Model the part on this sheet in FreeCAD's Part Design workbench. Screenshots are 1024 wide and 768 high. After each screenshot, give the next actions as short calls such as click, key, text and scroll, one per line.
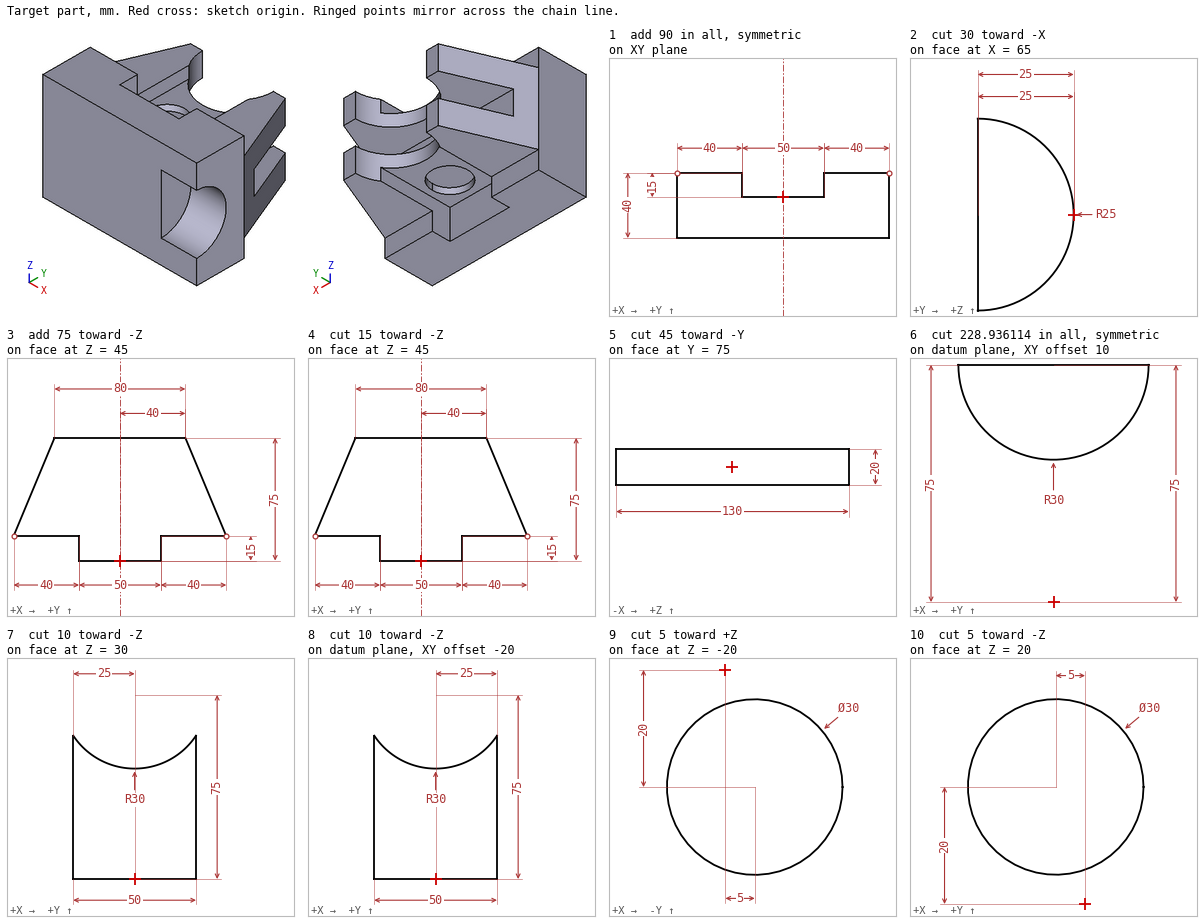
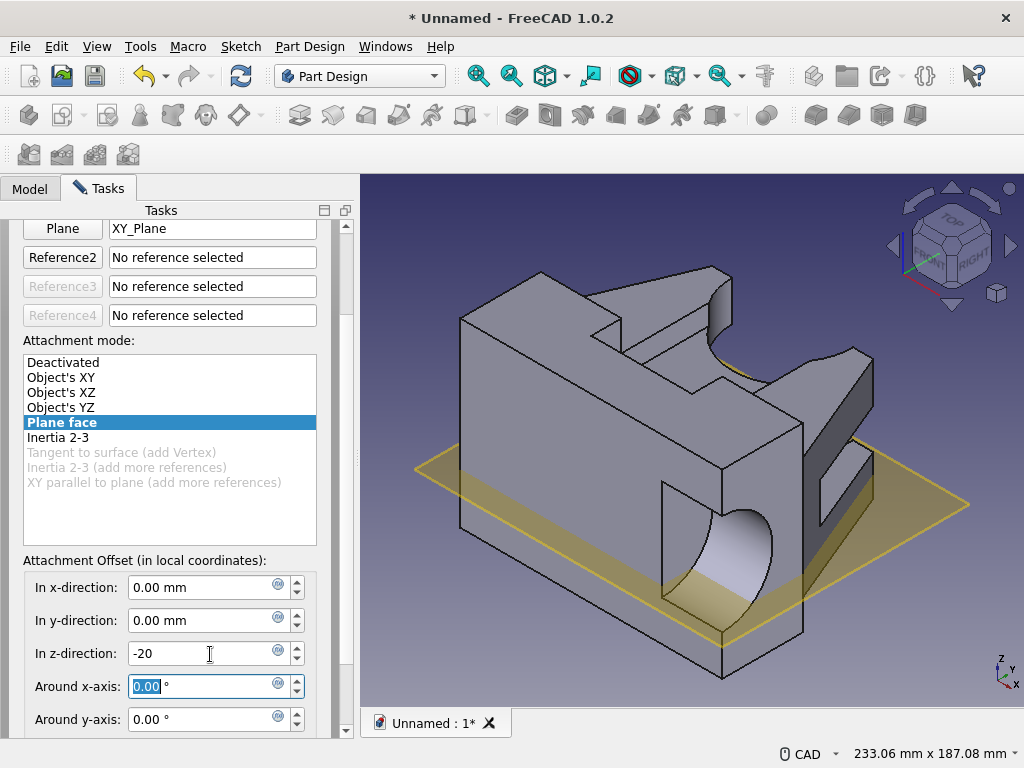
scroll(346, 479, up, 3)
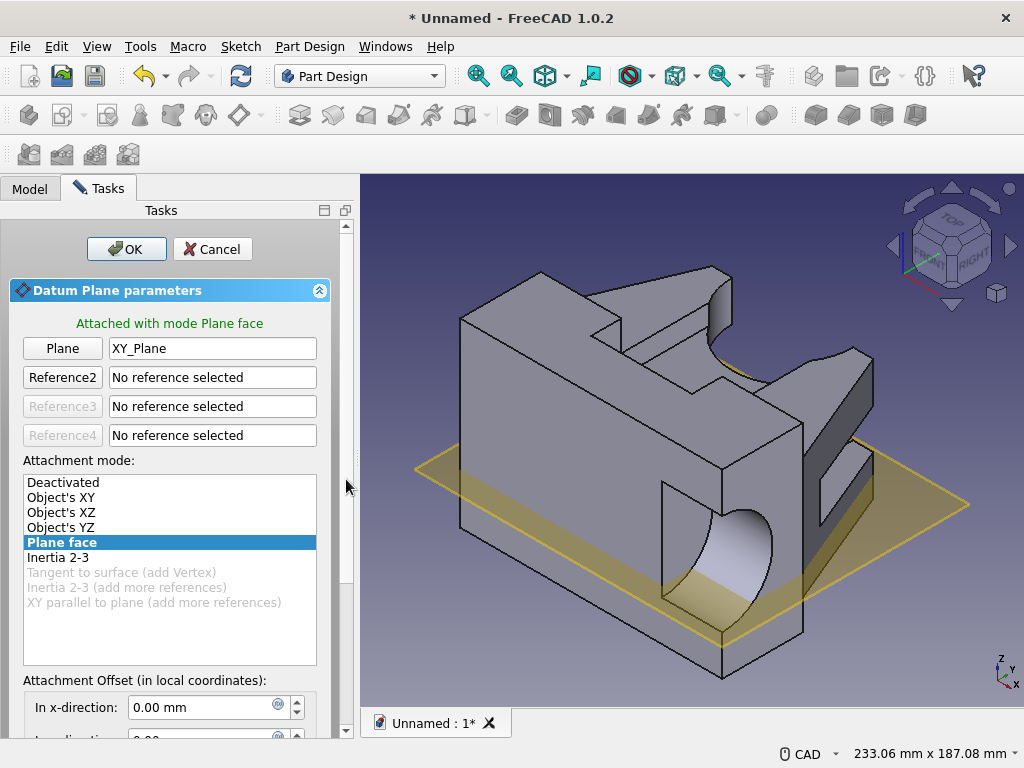
click(127, 249)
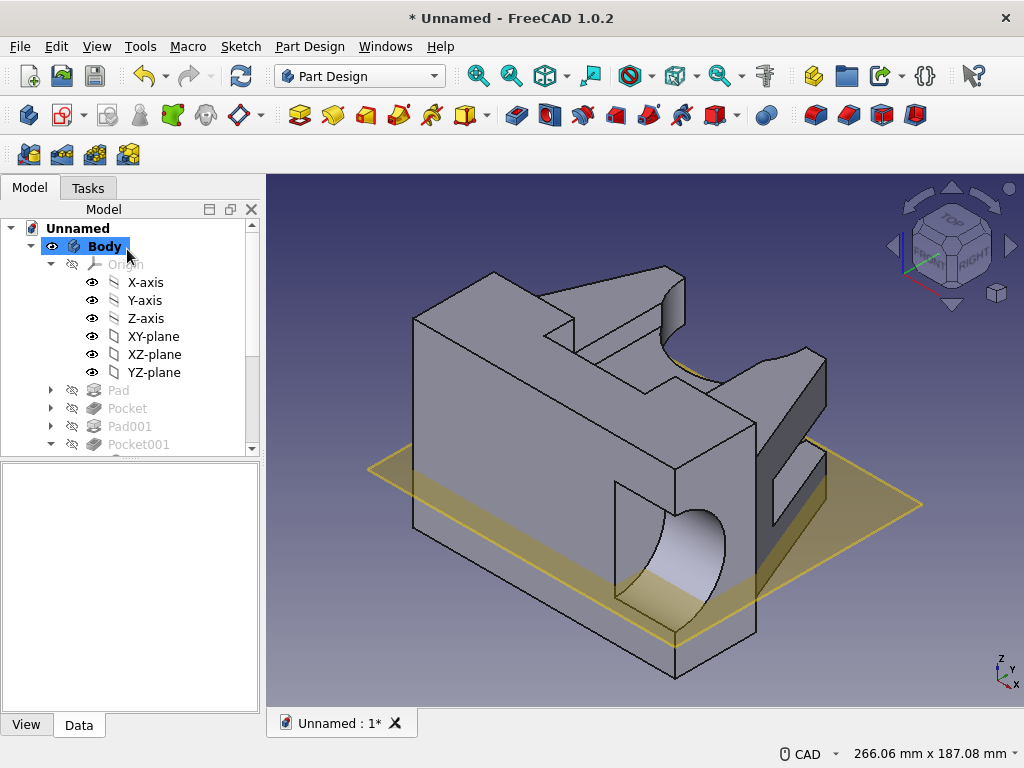
scroll(101, 332, down, 3)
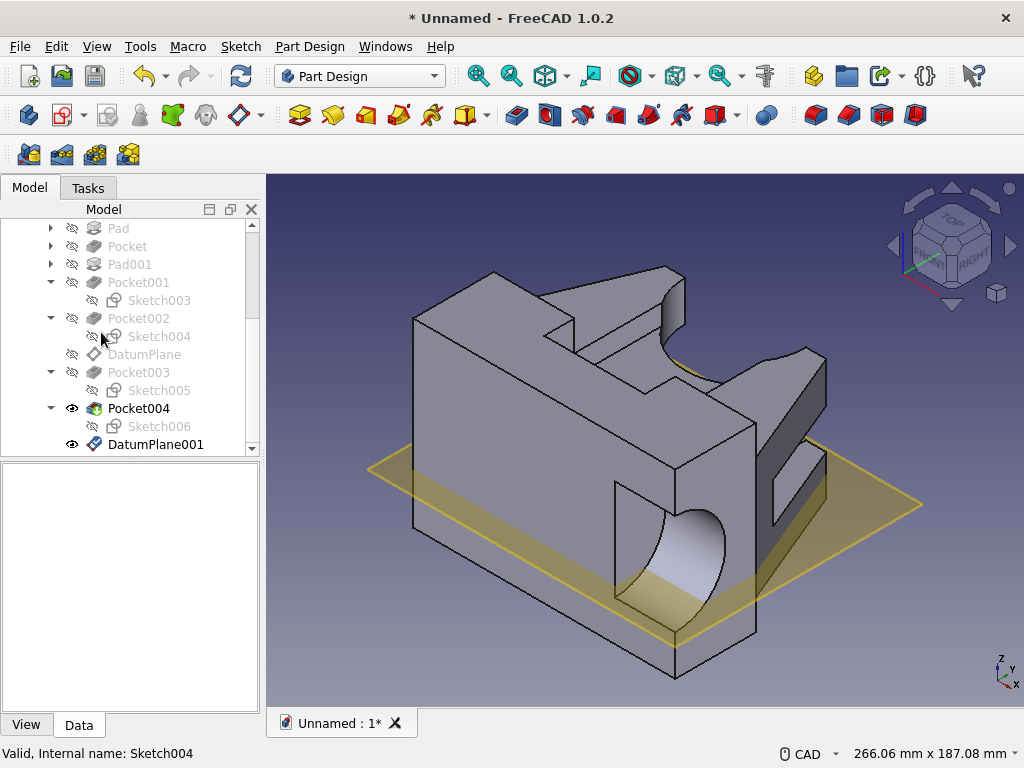
click(117, 444)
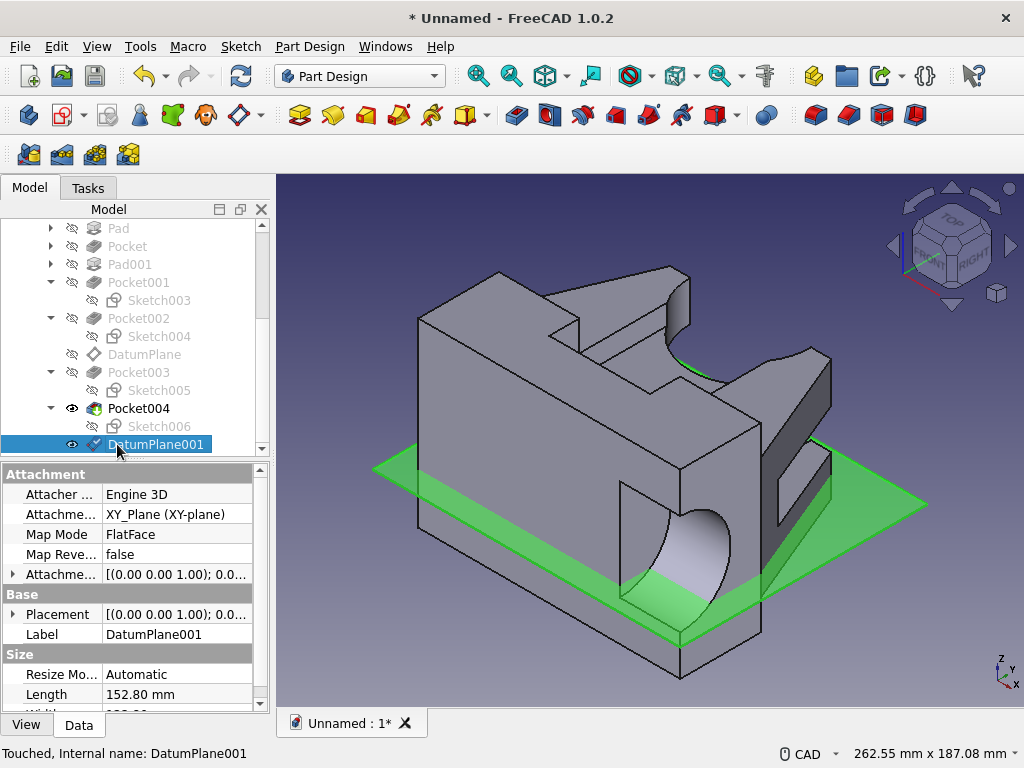
click(62, 116)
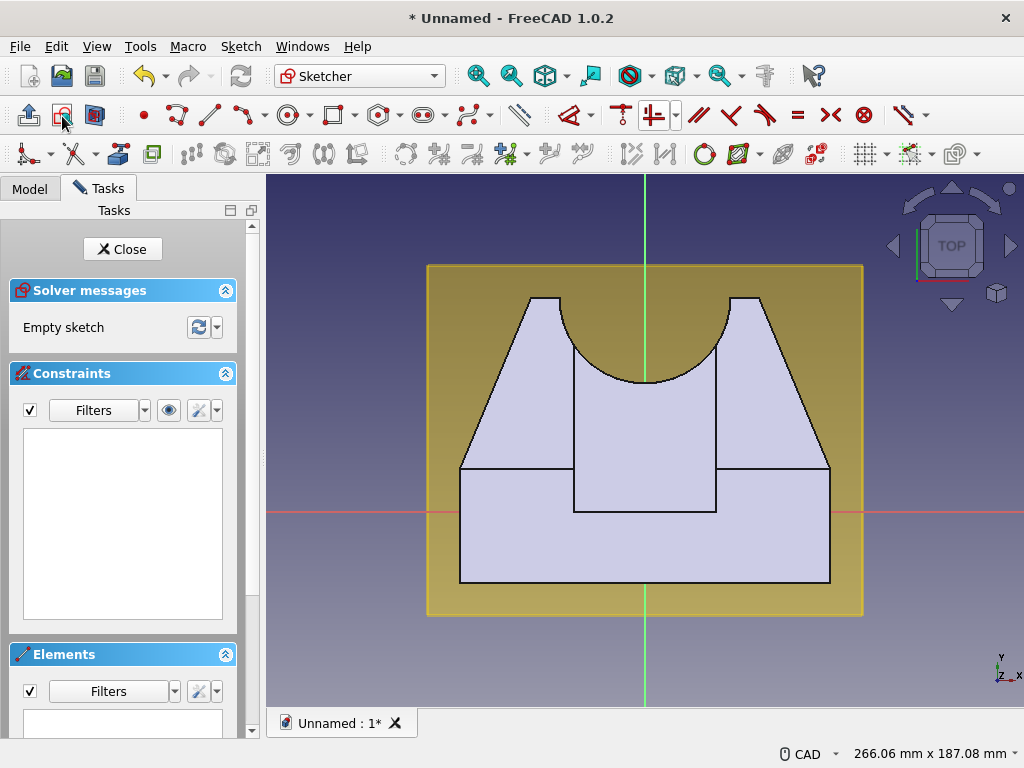
click(95, 116)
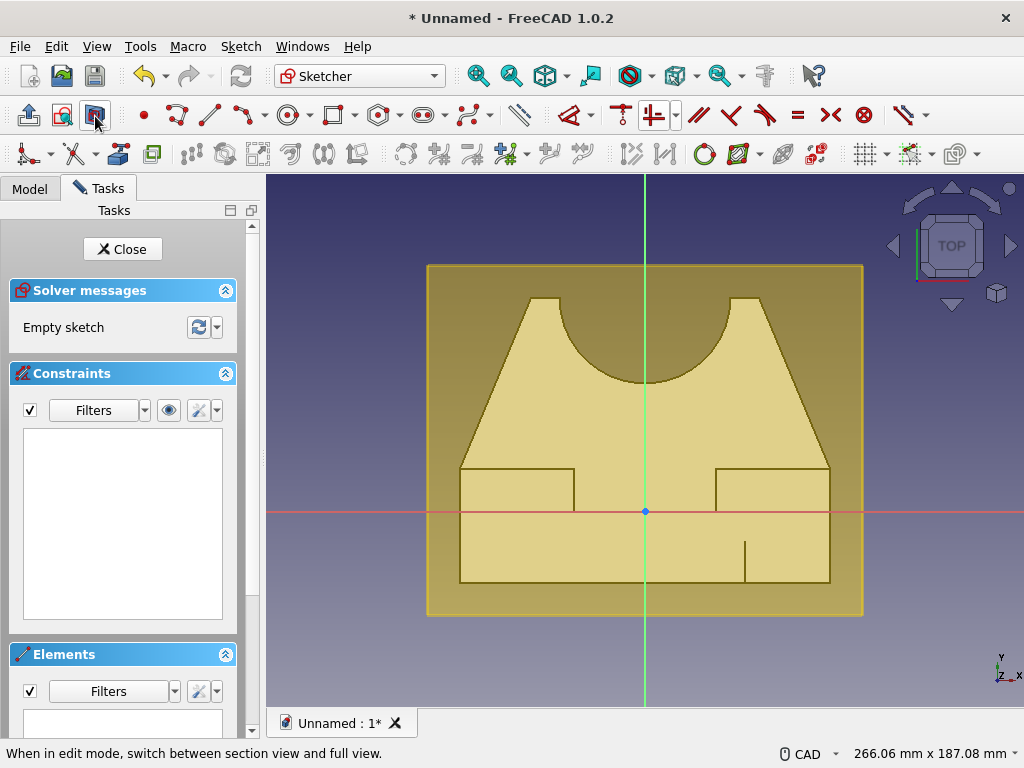
scroll(701, 419, up, 4)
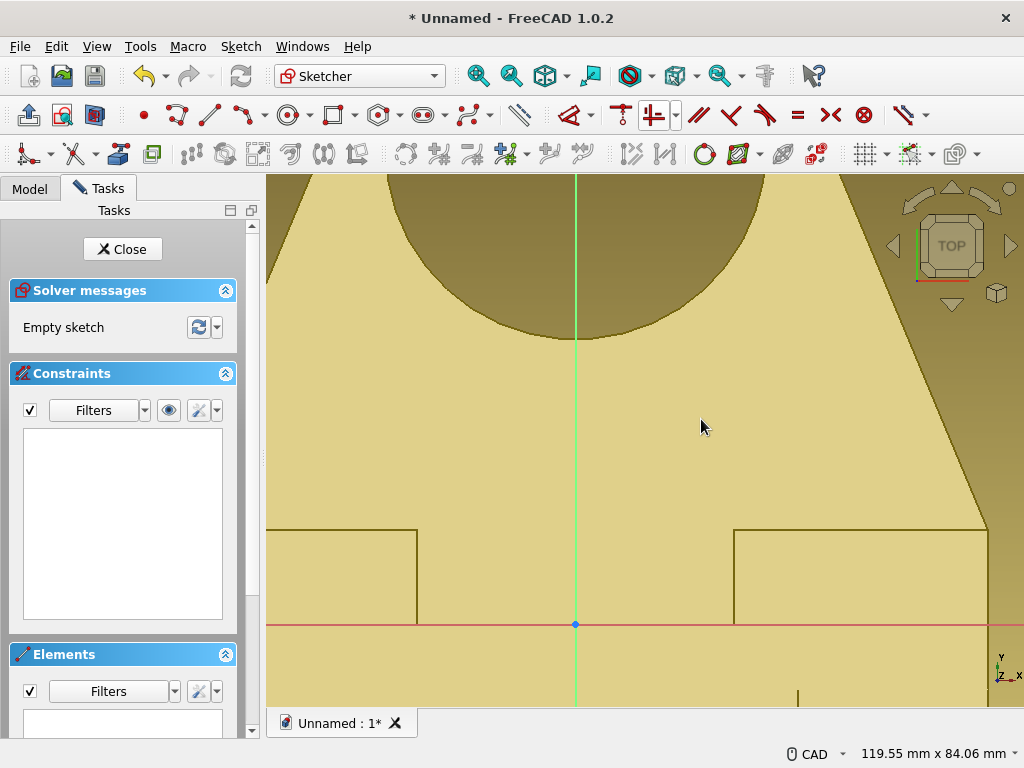
key(g)
key(m)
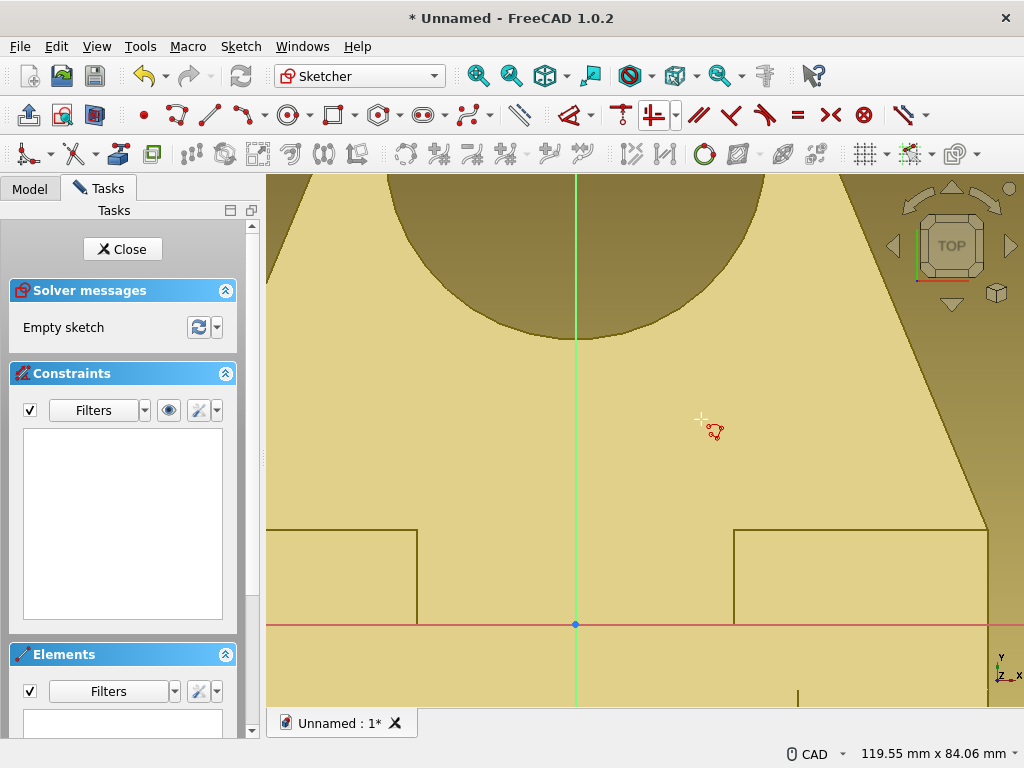
click(734, 254)
click(734, 625)
click(417, 616)
click(417, 254)
right_click(417, 254)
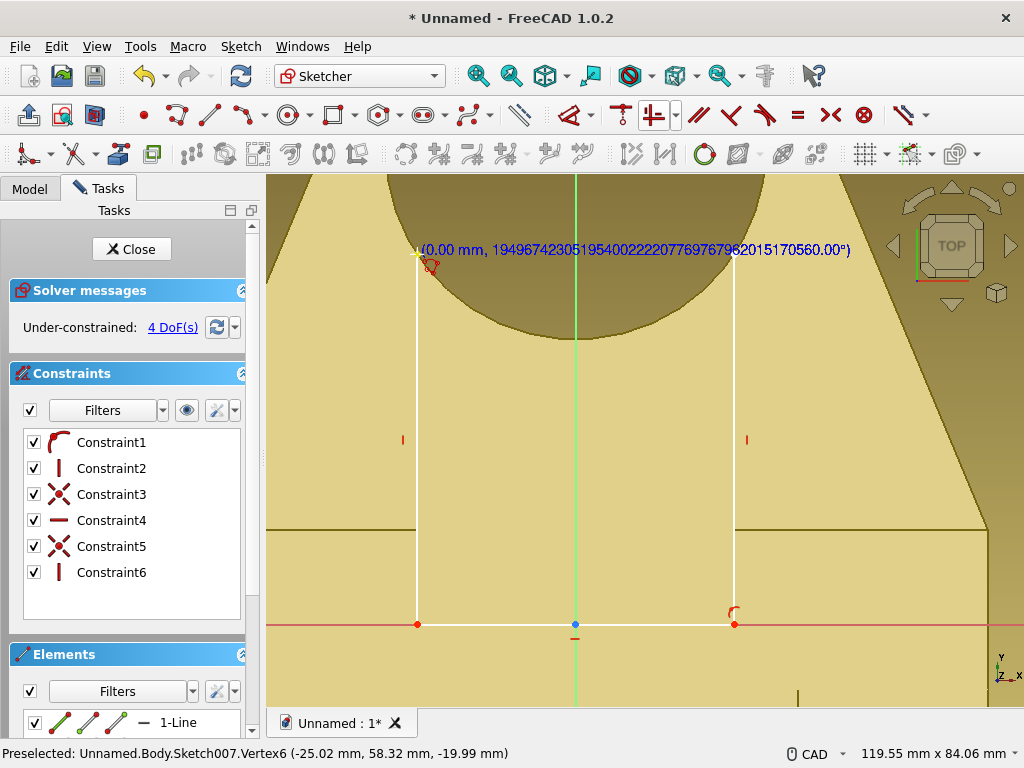
key(g)
key(3)
key(a)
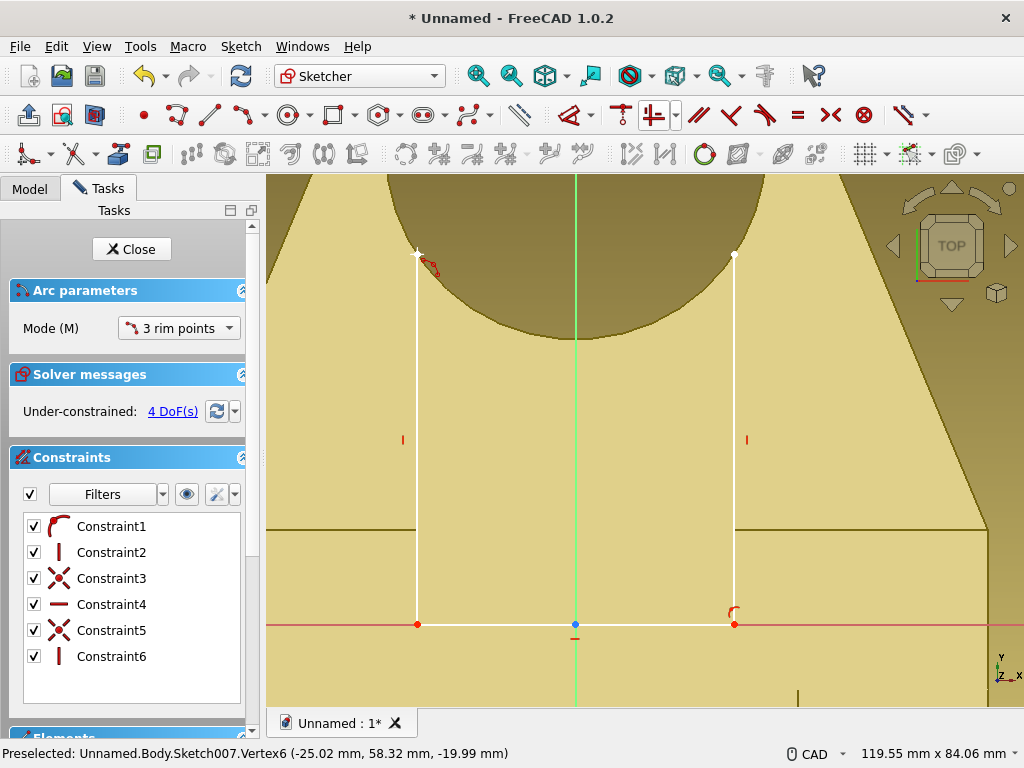
click(417, 255)
click(734, 255)
click(538, 336)
key(Escape)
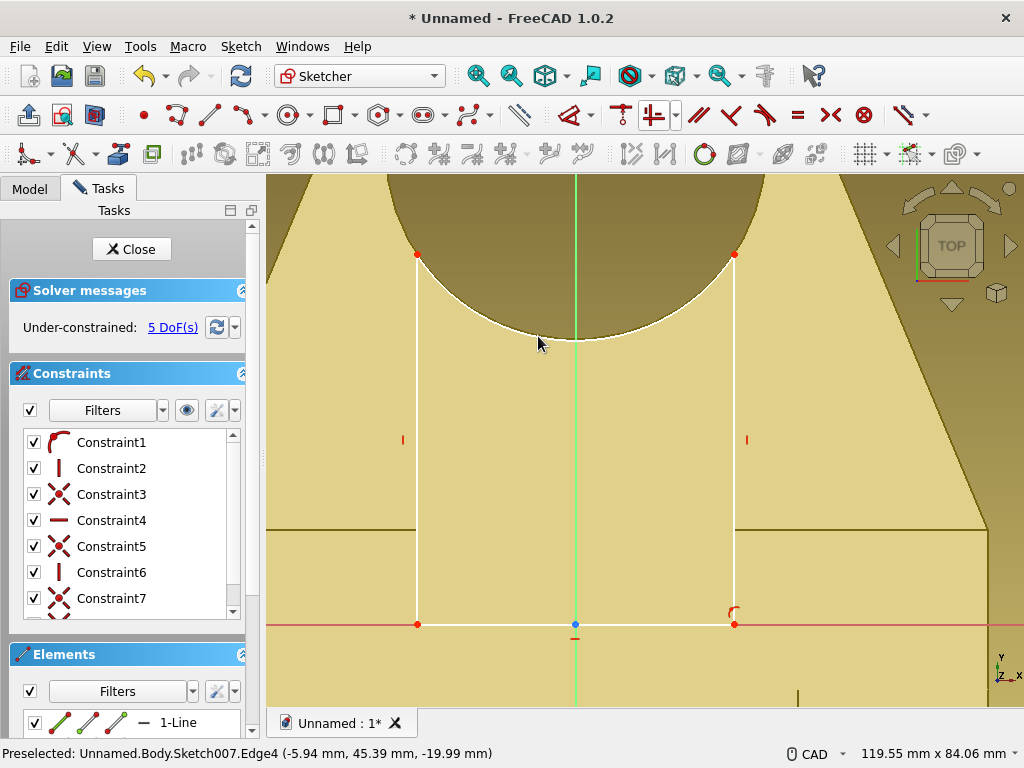
scroll(578, 547, down, 2)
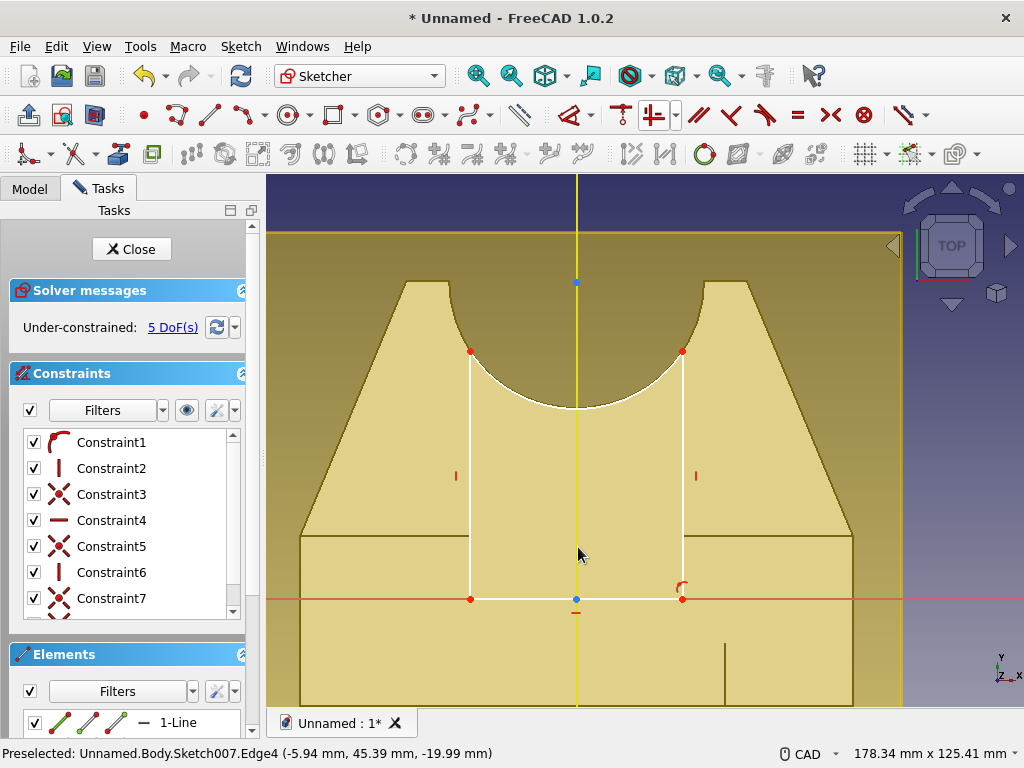
click(576, 282)